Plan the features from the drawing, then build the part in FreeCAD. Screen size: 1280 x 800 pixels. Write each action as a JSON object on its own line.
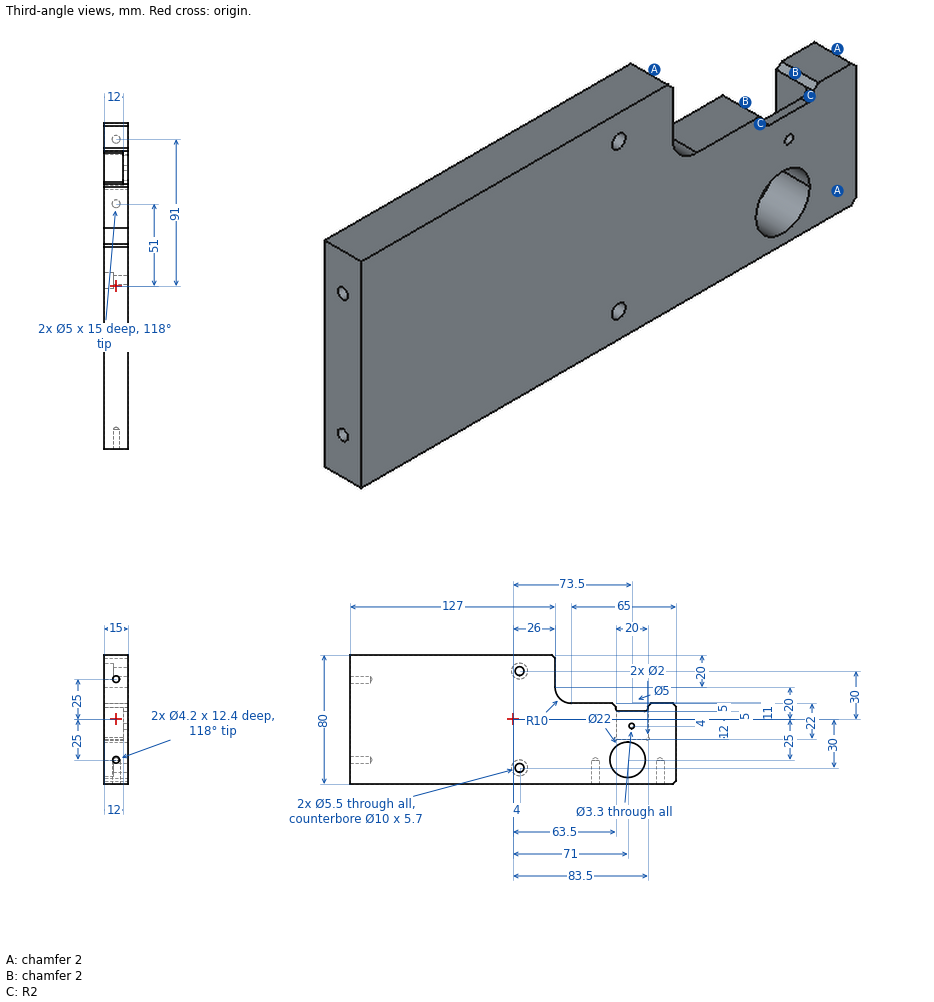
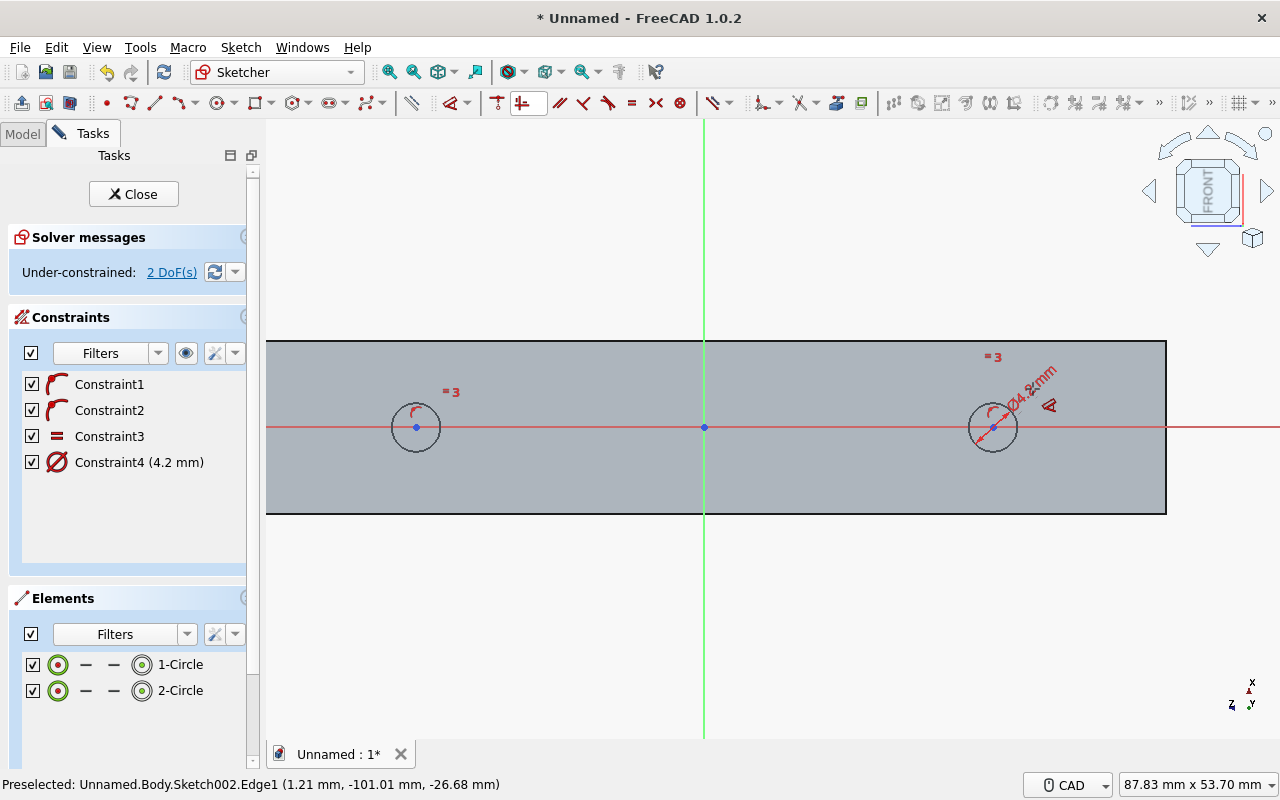
{"action": "left_click", "coordinate": [993, 427]}
{"action": "left_click", "coordinate": [849, 461]}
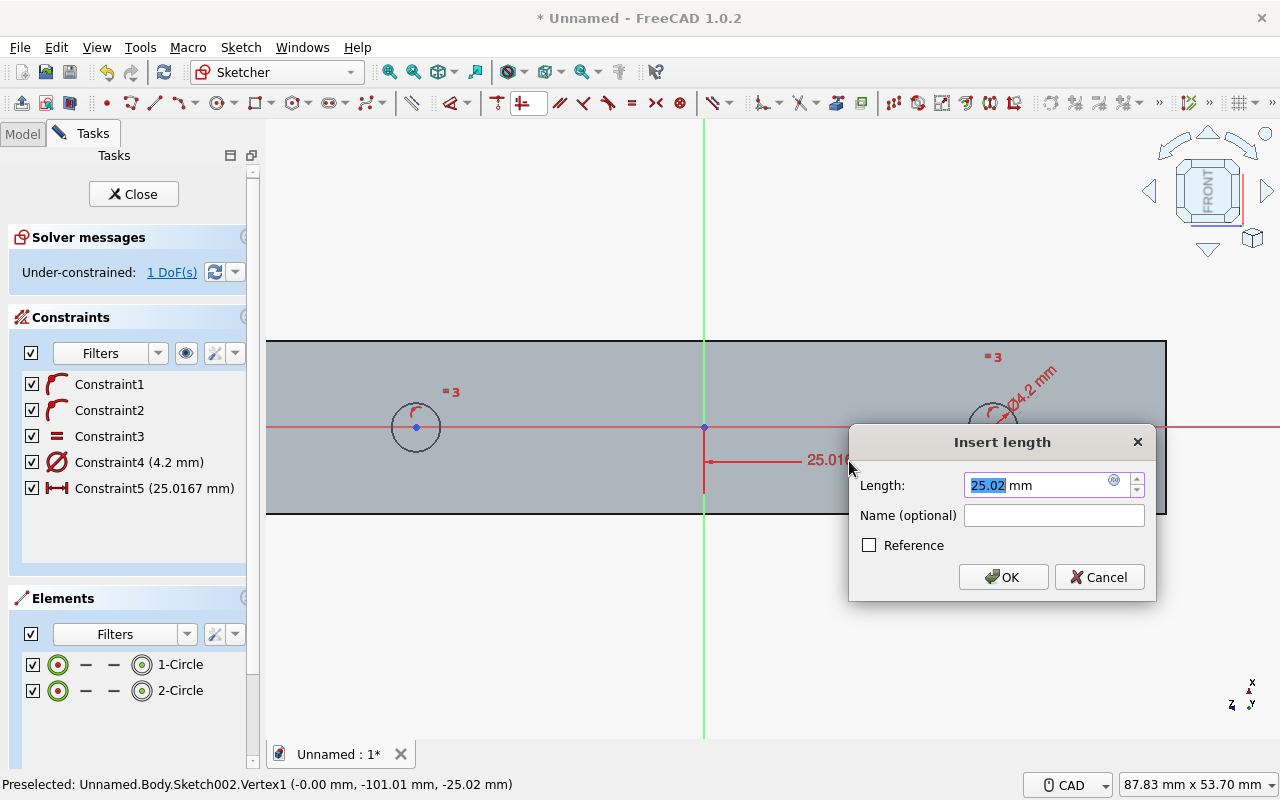
{"action": "type", "text": "25"}
{"action": "key", "text": "Return"}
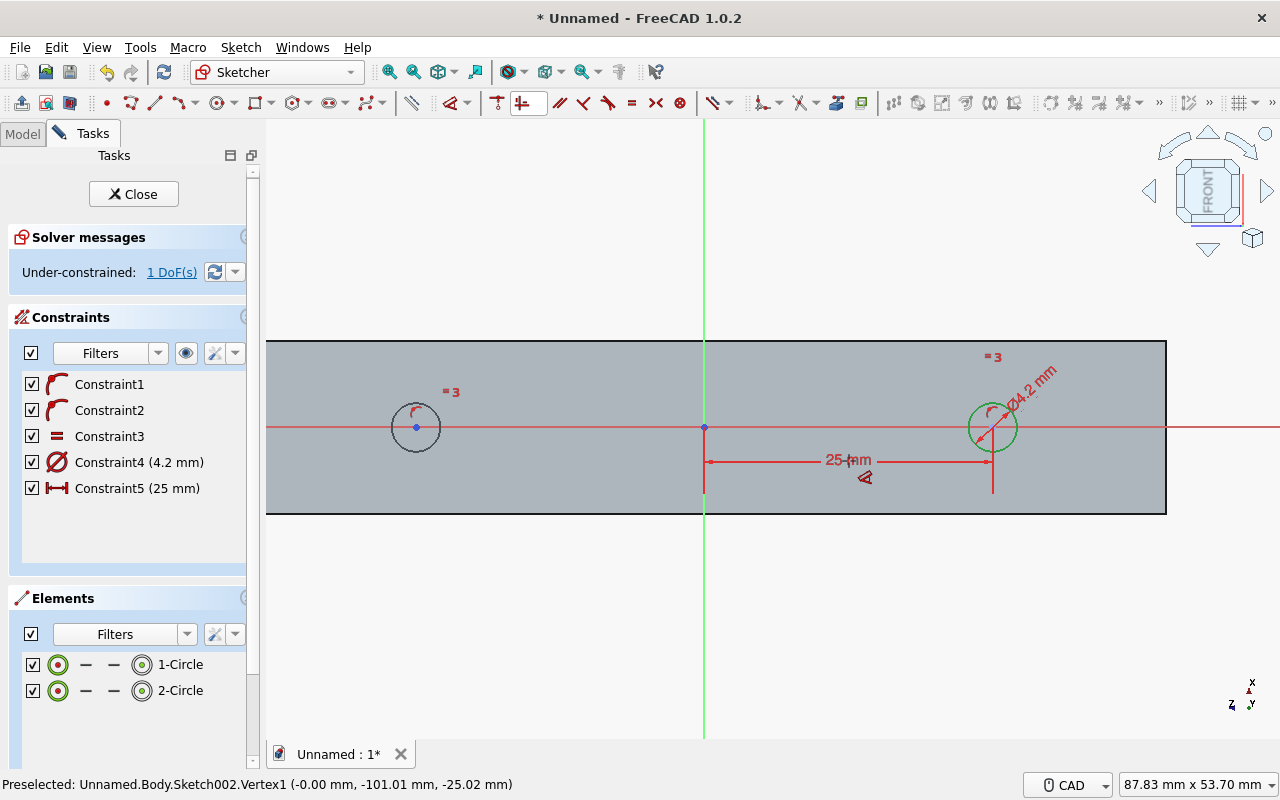
{"action": "left_click", "coordinate": [416, 427]}
{"action": "left_click", "coordinate": [560, 461]}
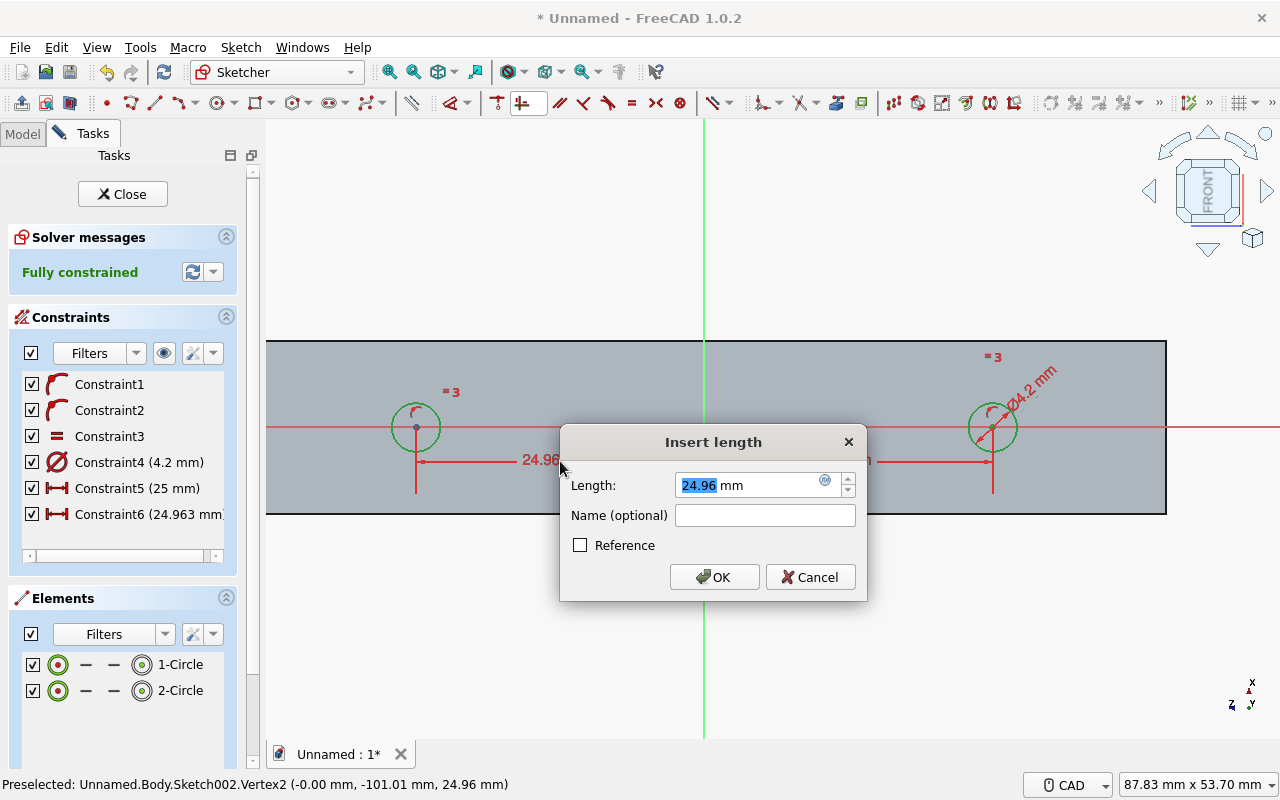
{"action": "type", "text": "25"}
{"action": "key", "text": "Return"}
{"action": "key", "text": "Escape"}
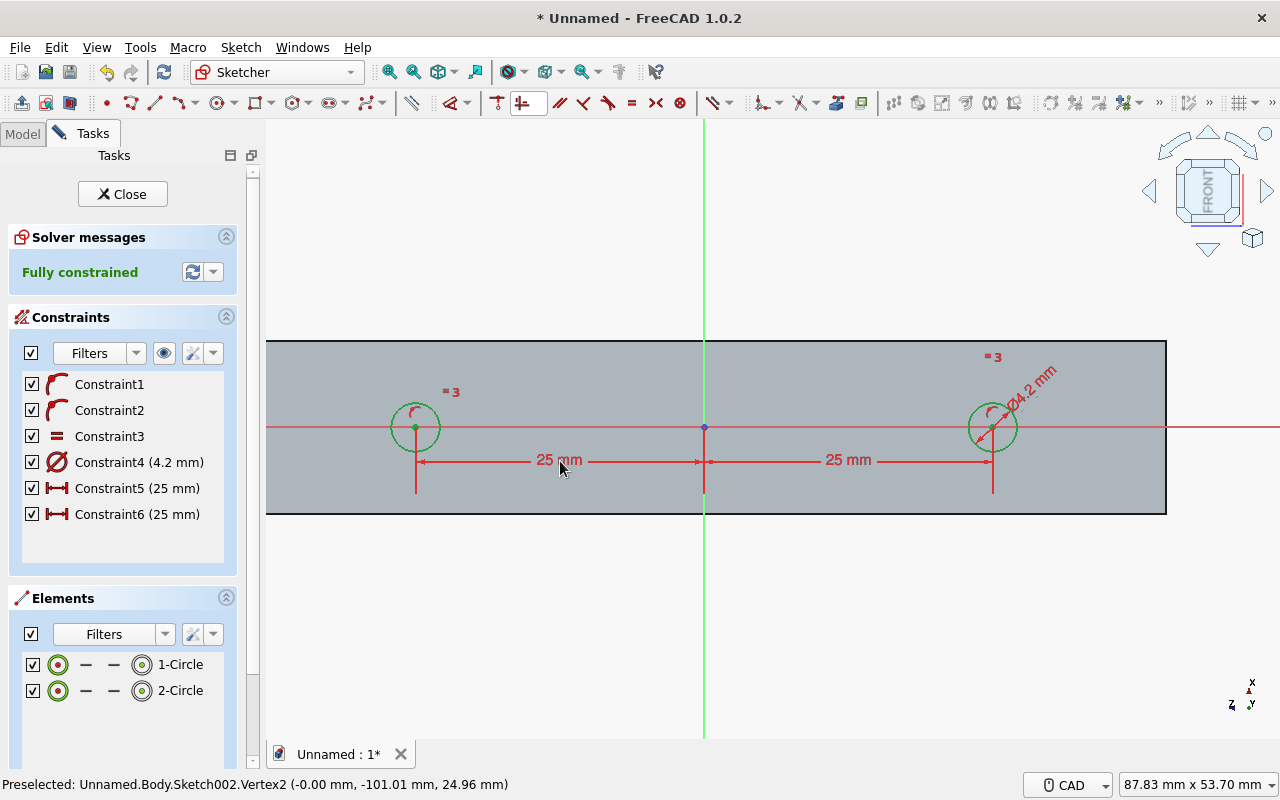
{"action": "left_click", "coordinate": [123, 194]}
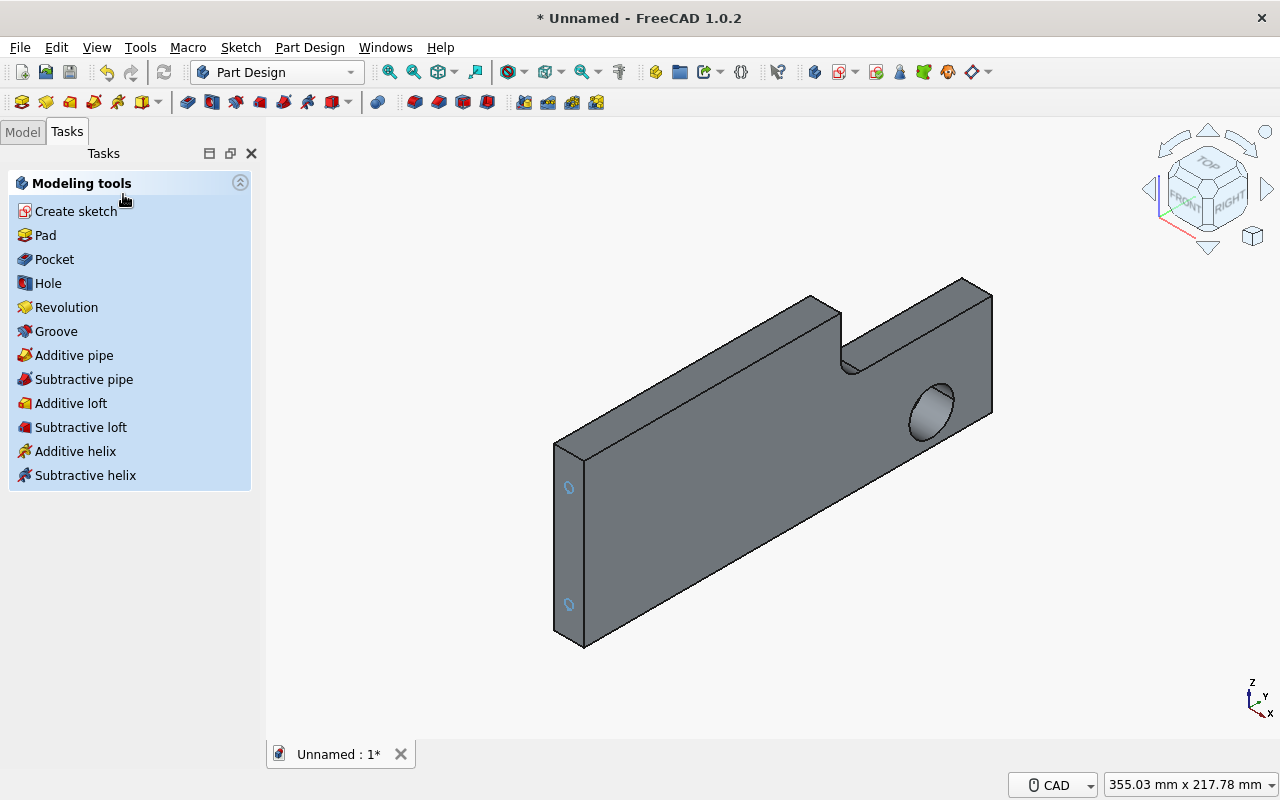
{"action": "left_click", "coordinate": [212, 102]}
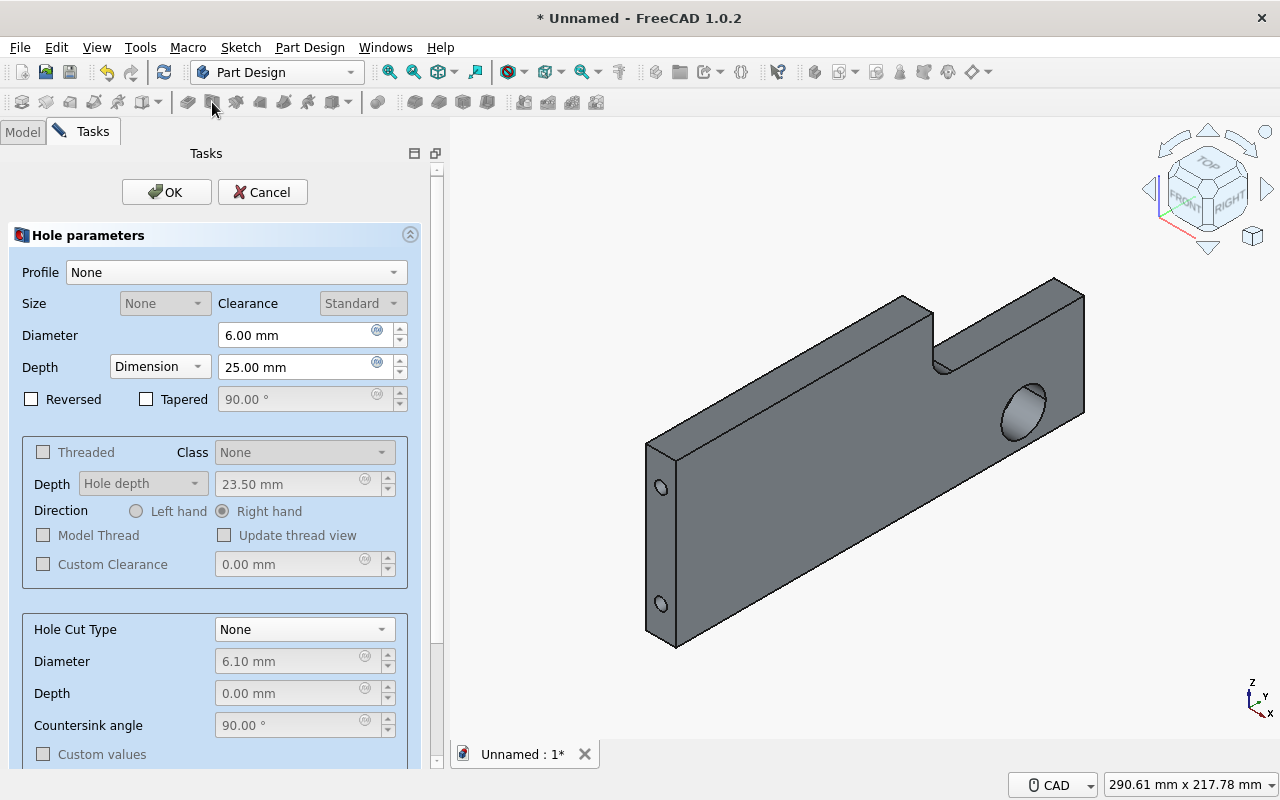
{"action": "triple_click", "coordinate": [305, 335]}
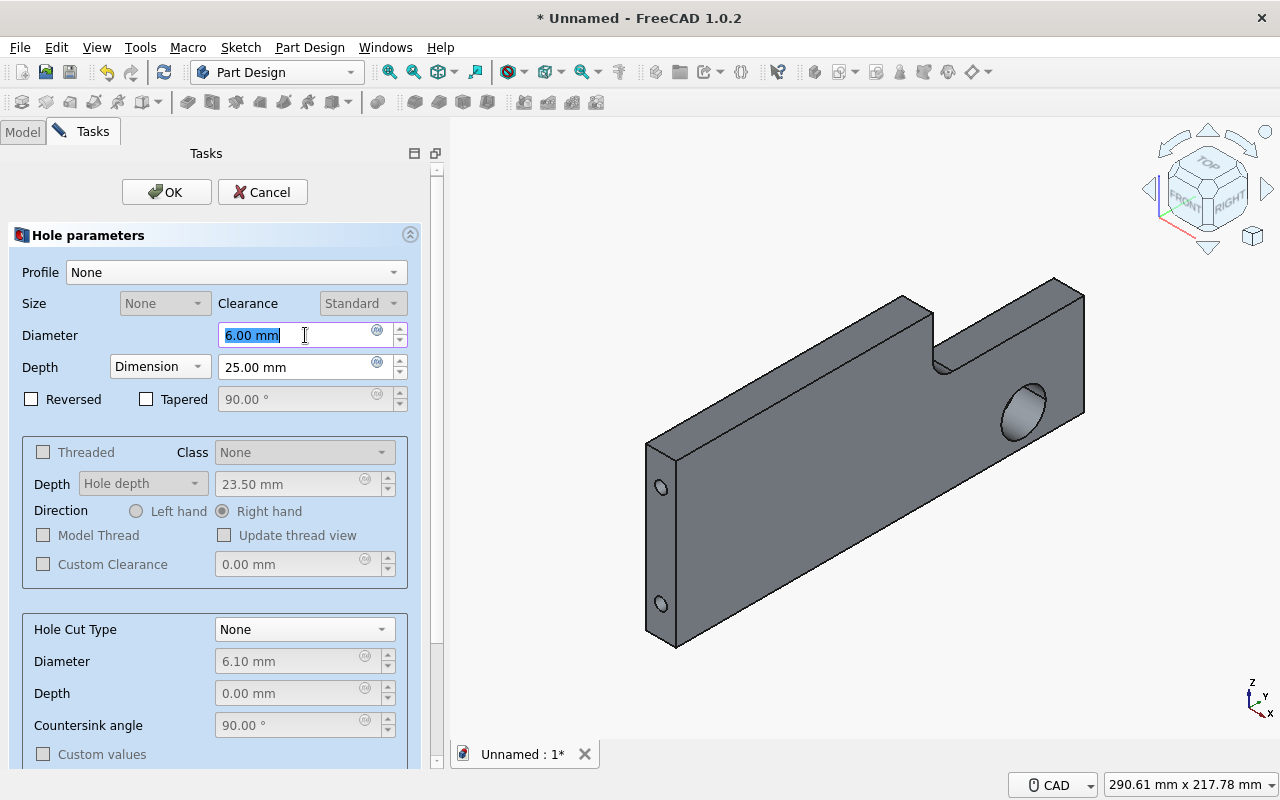
{"action": "type", "text": "4.2"}
{"action": "key", "text": "Tab"}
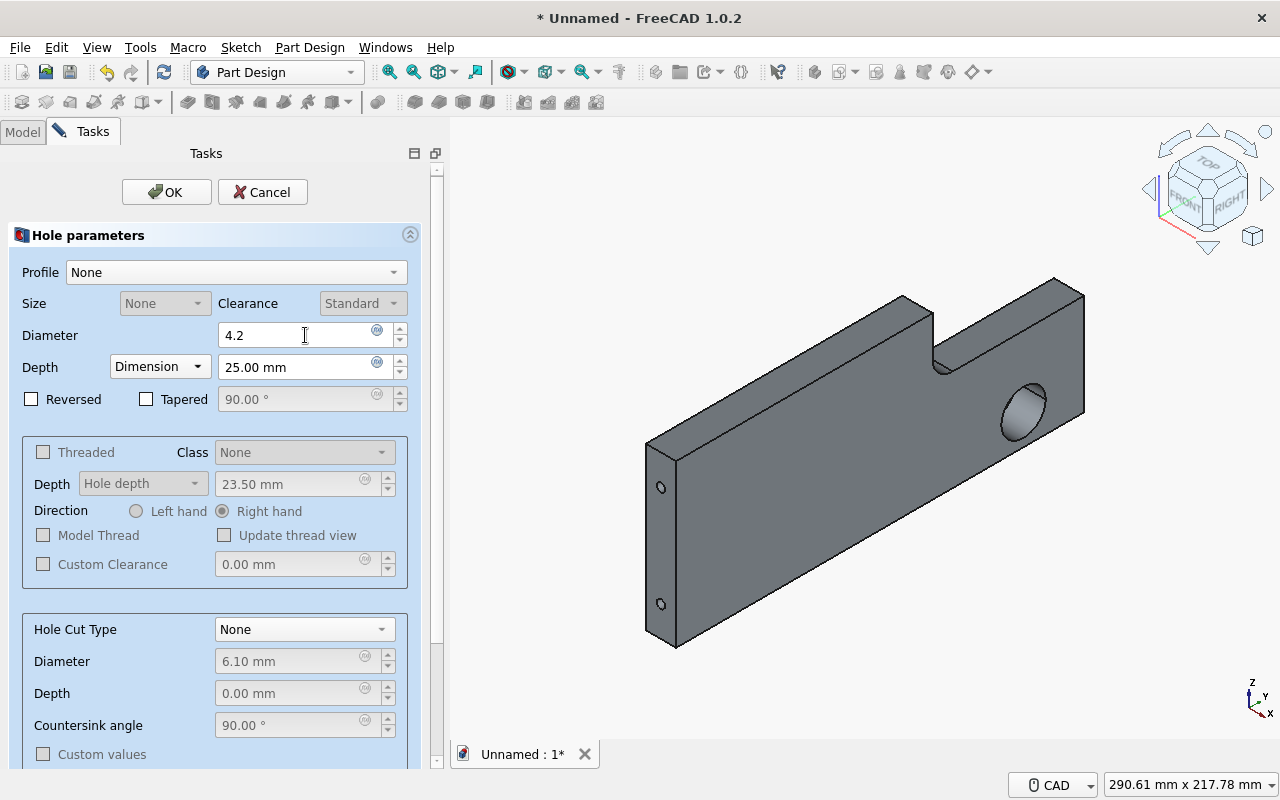
{"action": "triple_click", "coordinate": [305, 367]}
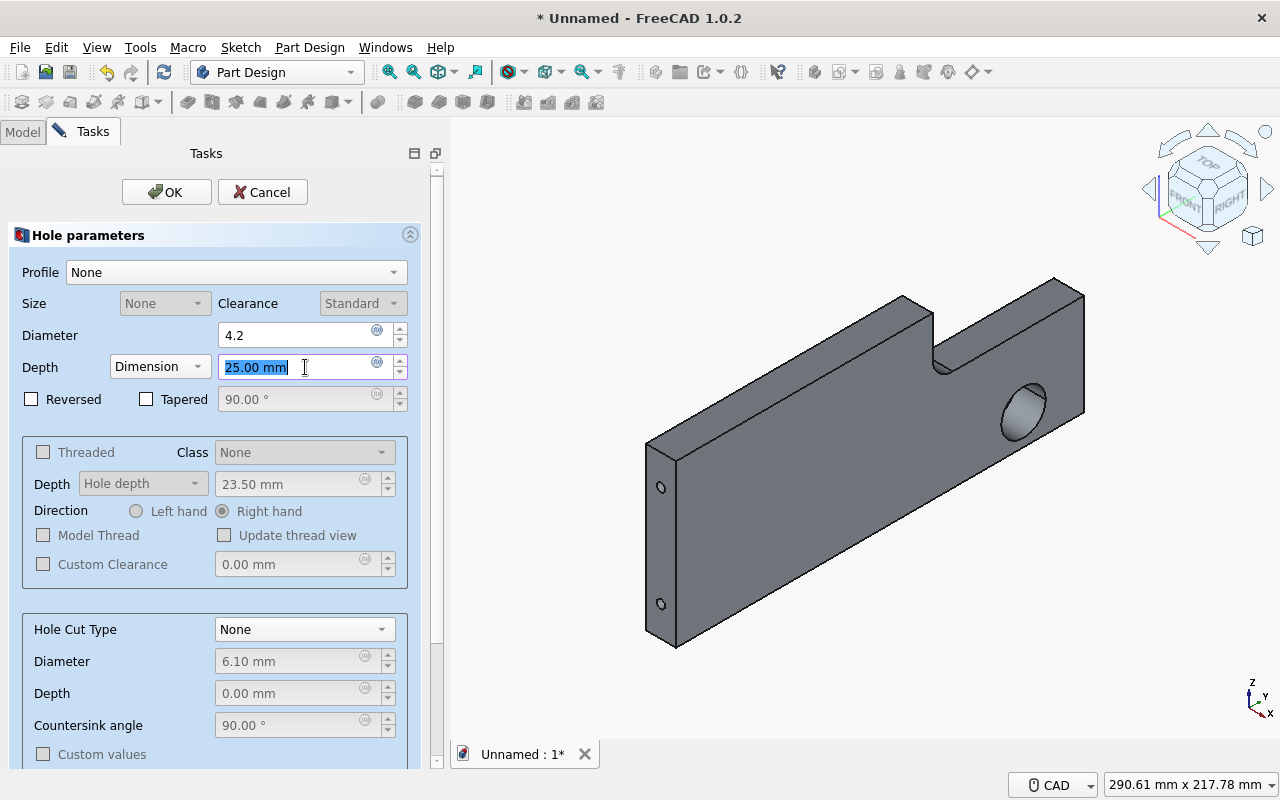
{"action": "type", "text": "12.4"}
{"action": "key", "text": "Tab"}